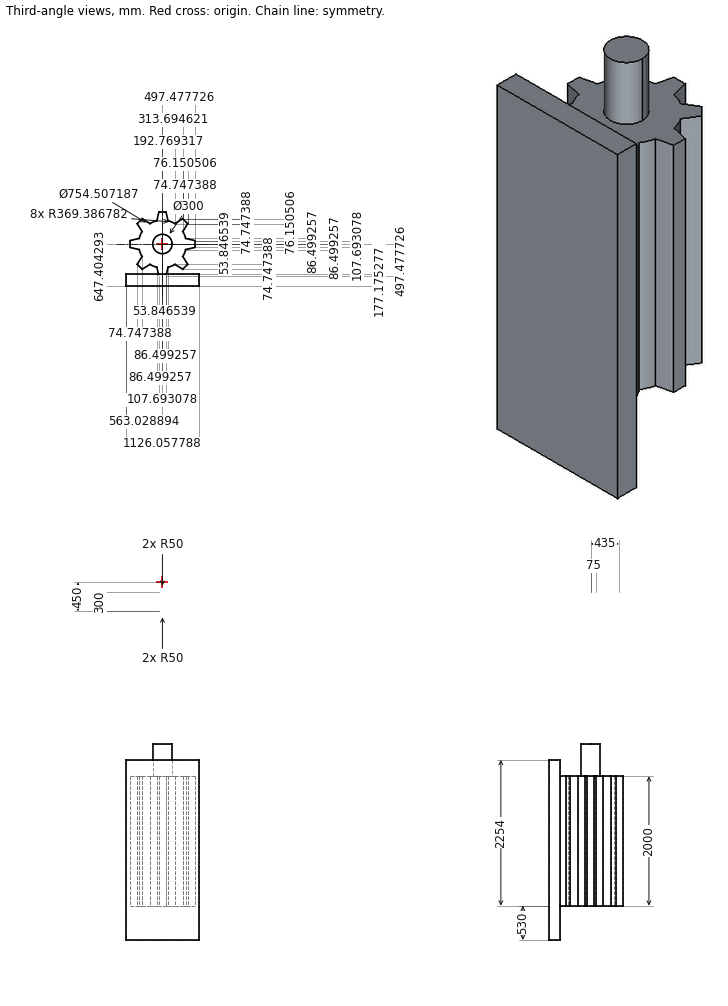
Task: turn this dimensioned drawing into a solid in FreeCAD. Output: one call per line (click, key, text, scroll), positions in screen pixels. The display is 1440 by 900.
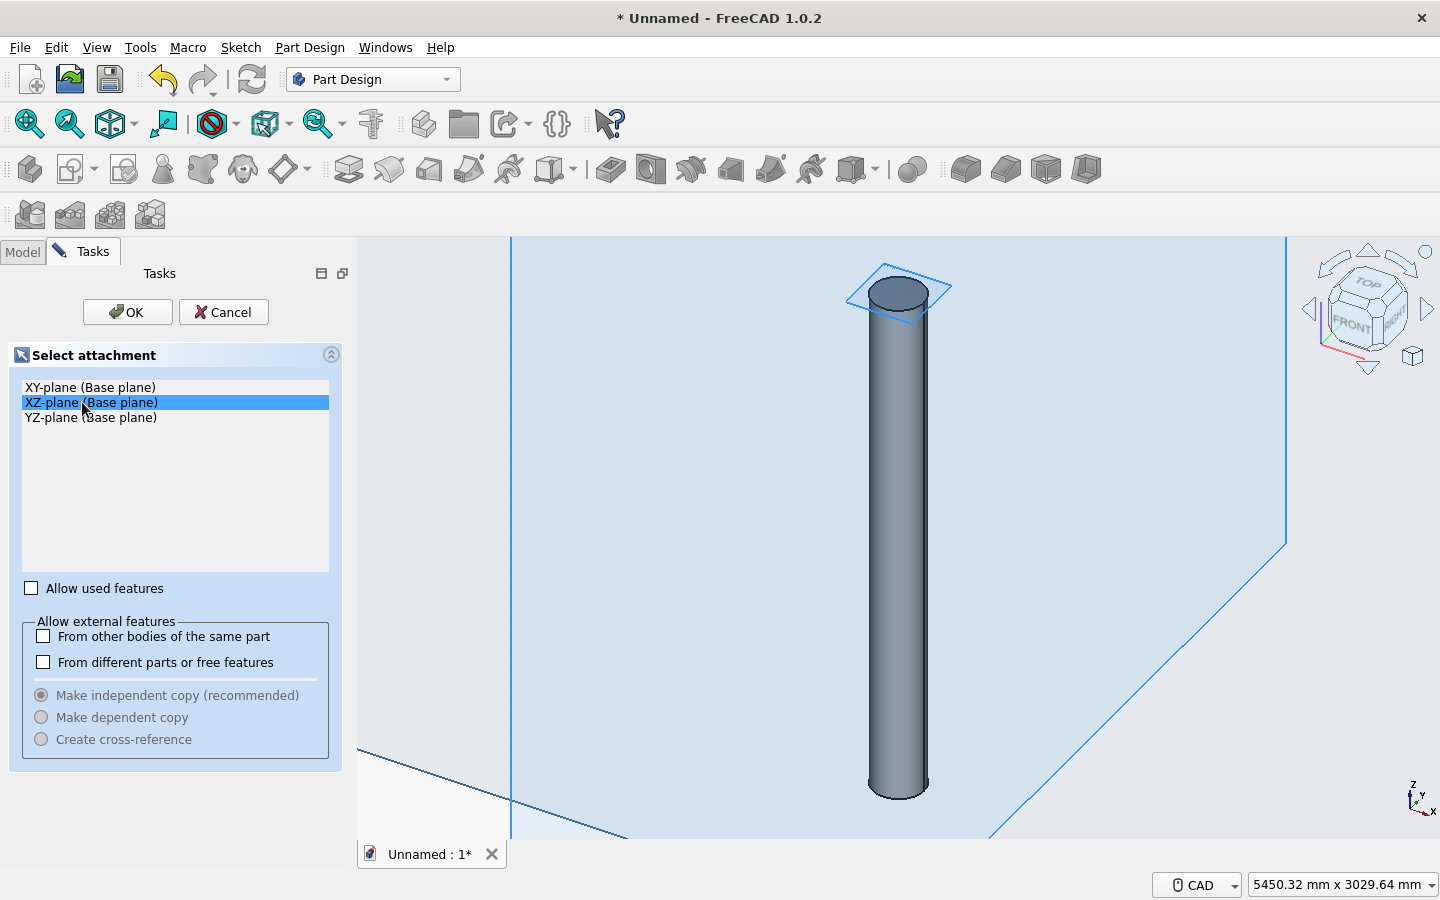
click(128, 312)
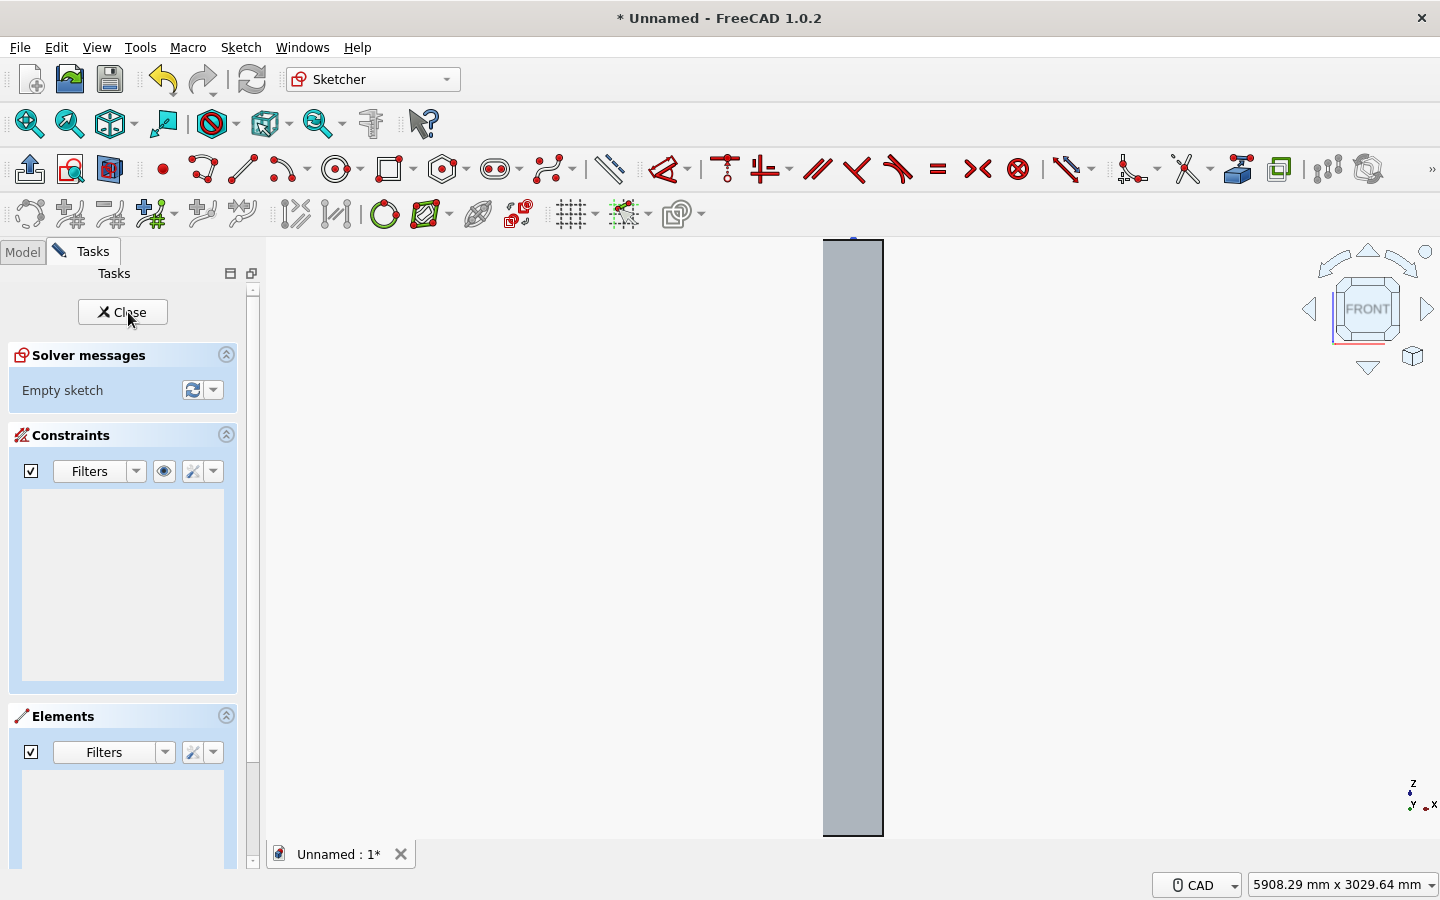
click(110, 170)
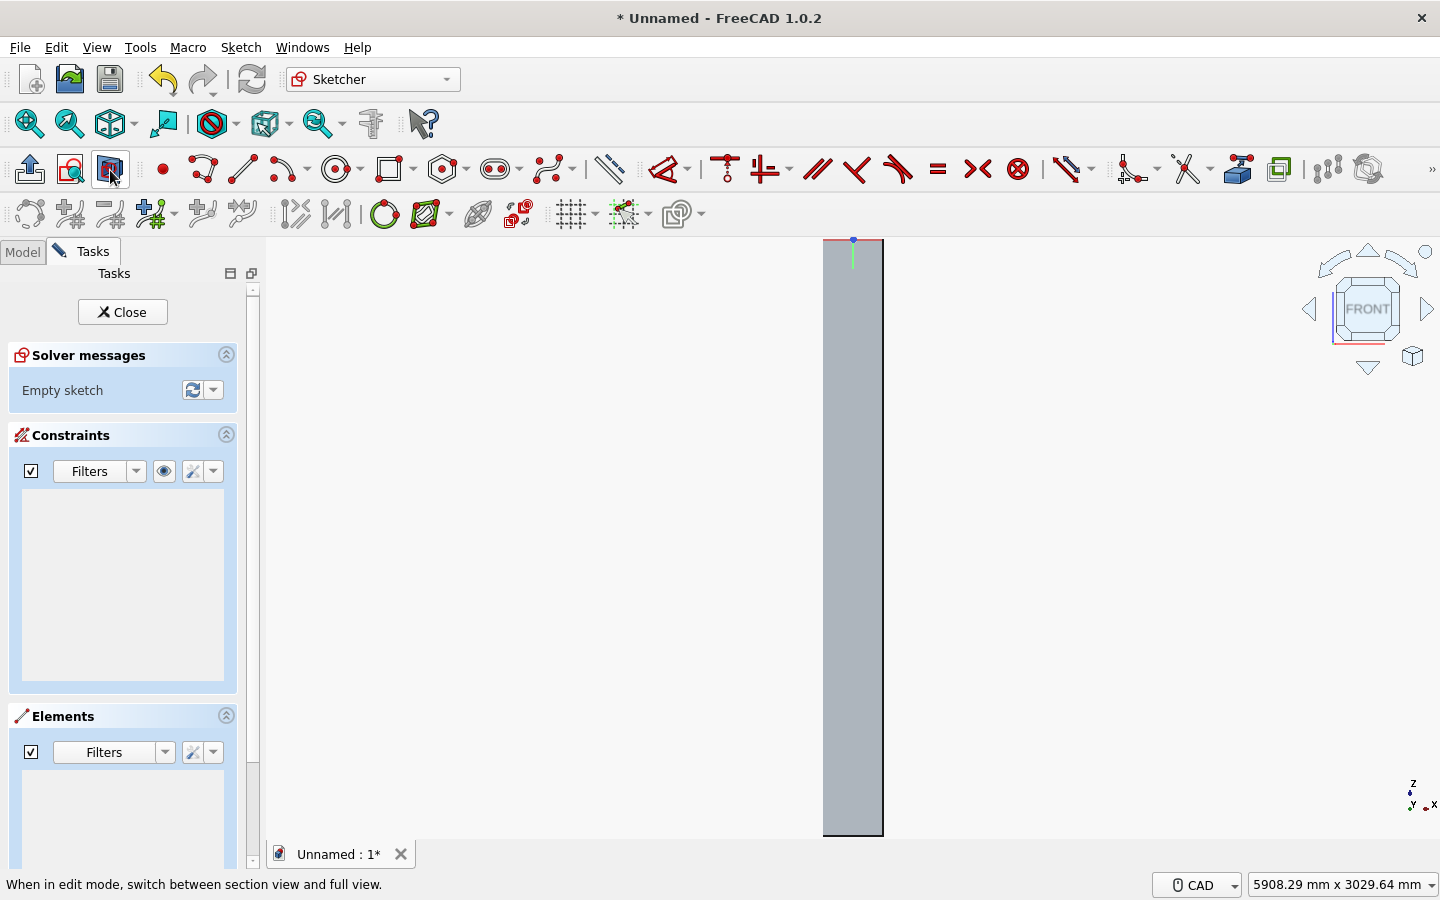
scroll(784, 538, down, 5)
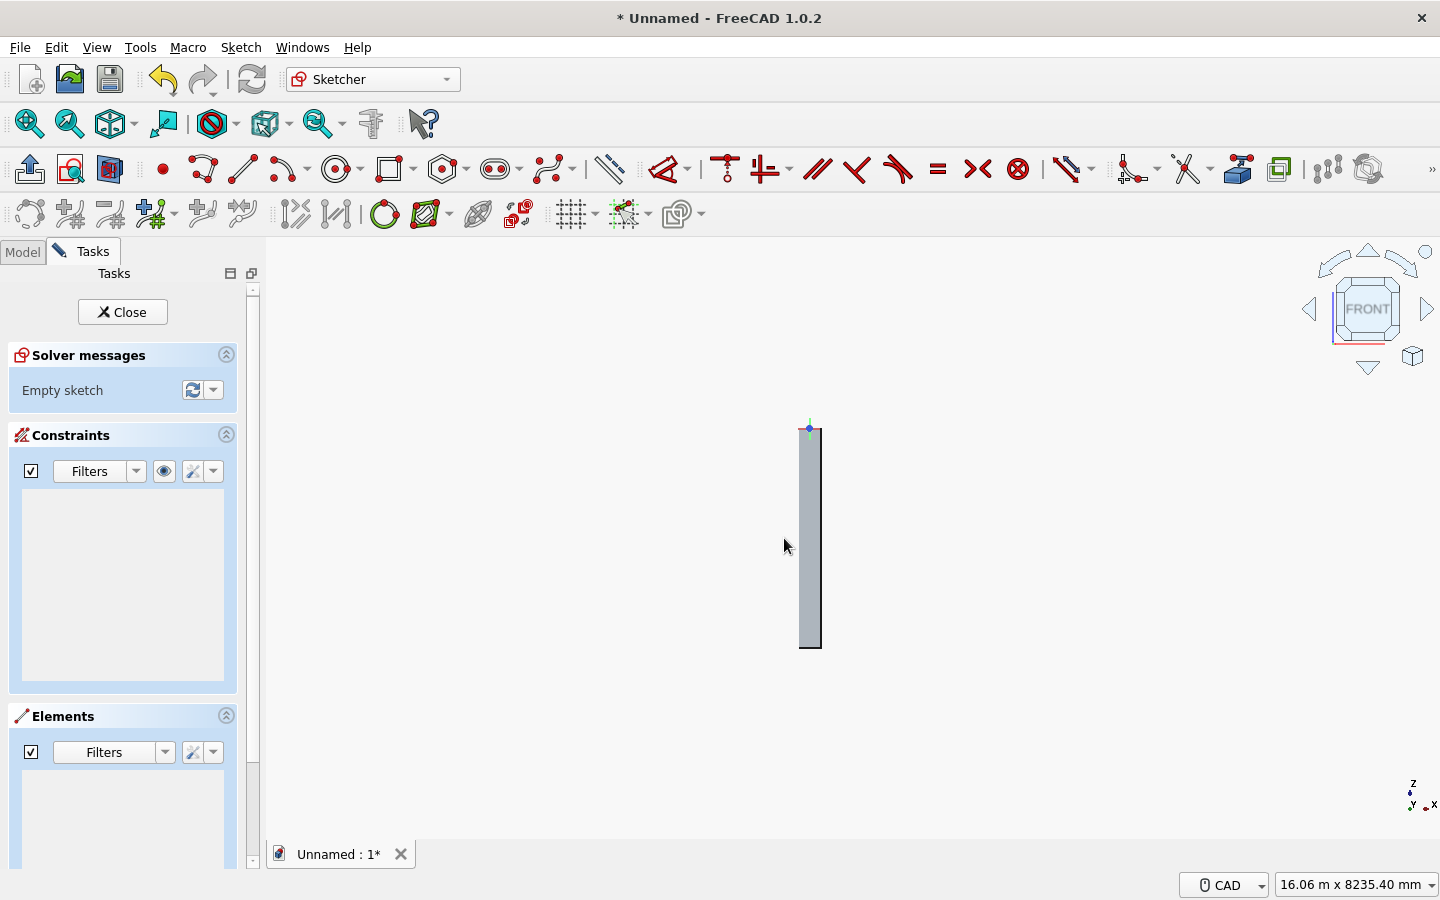
scroll(812, 438, up, 12)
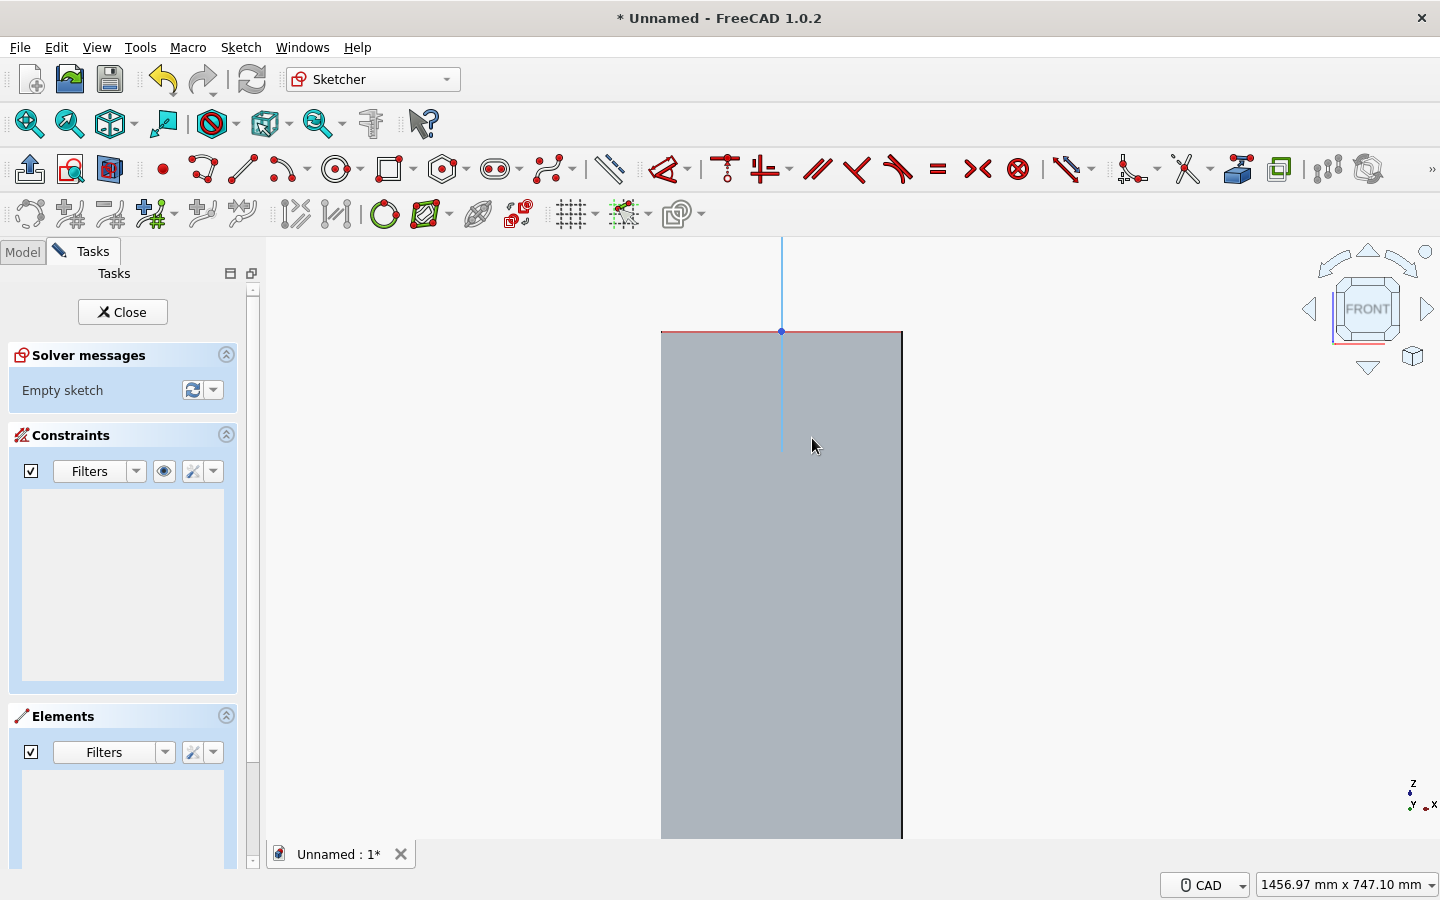
click(496, 170)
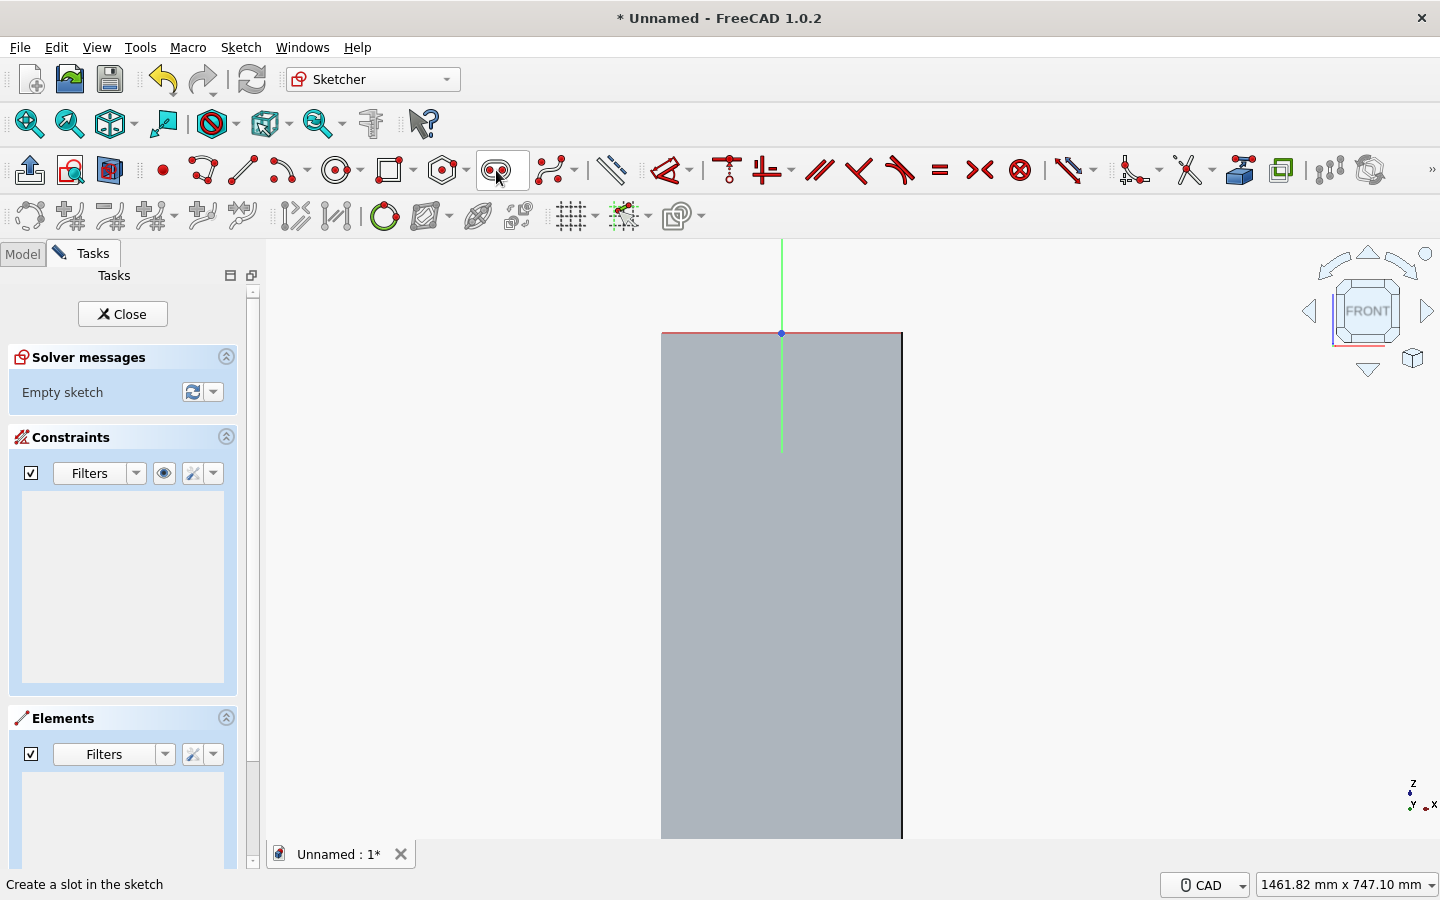
click(782, 695)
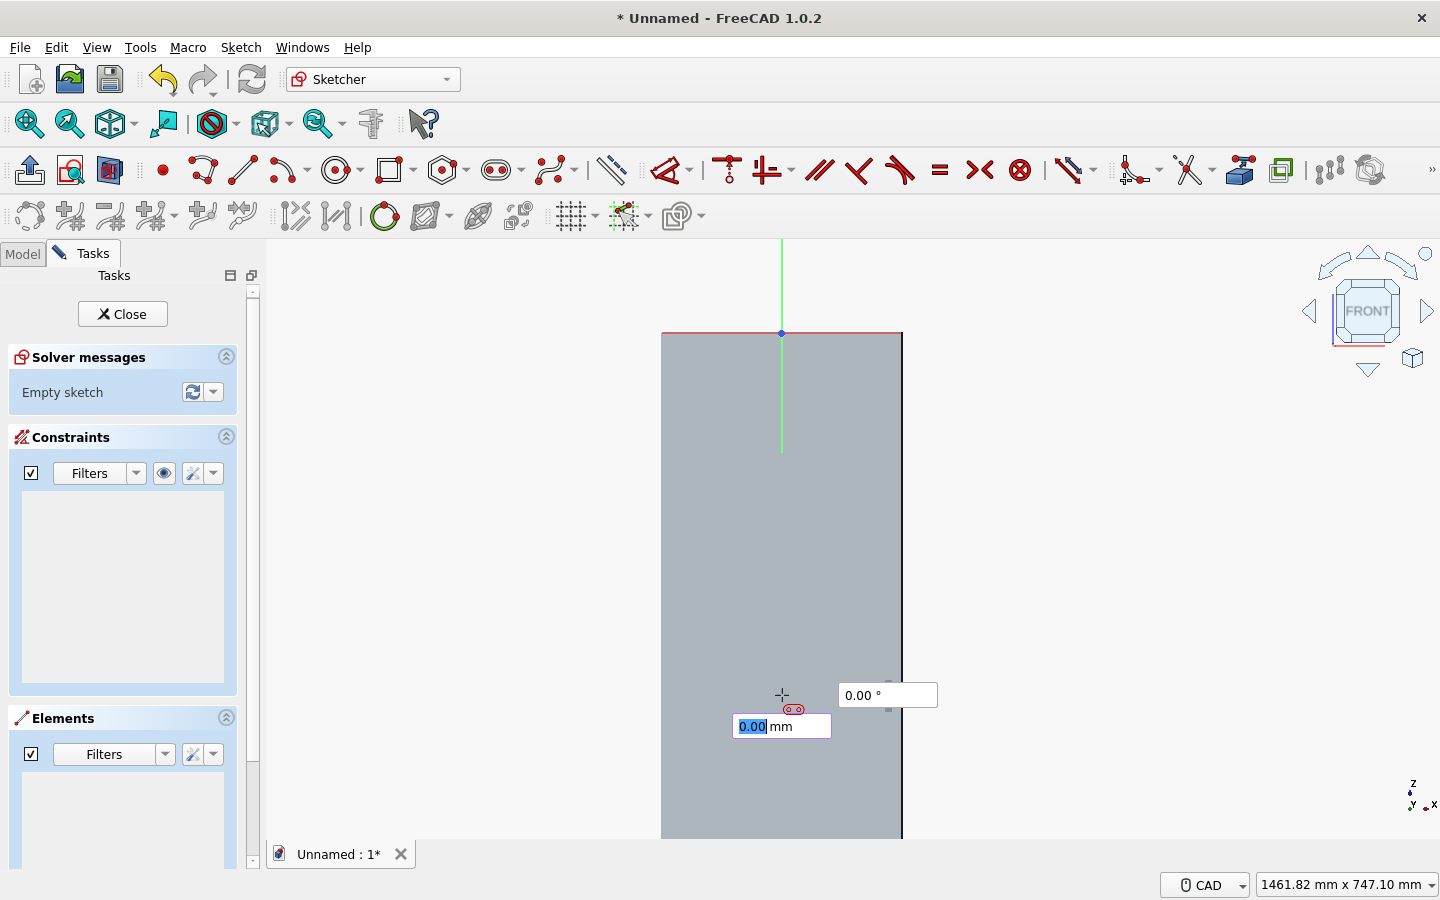
click(791, 454)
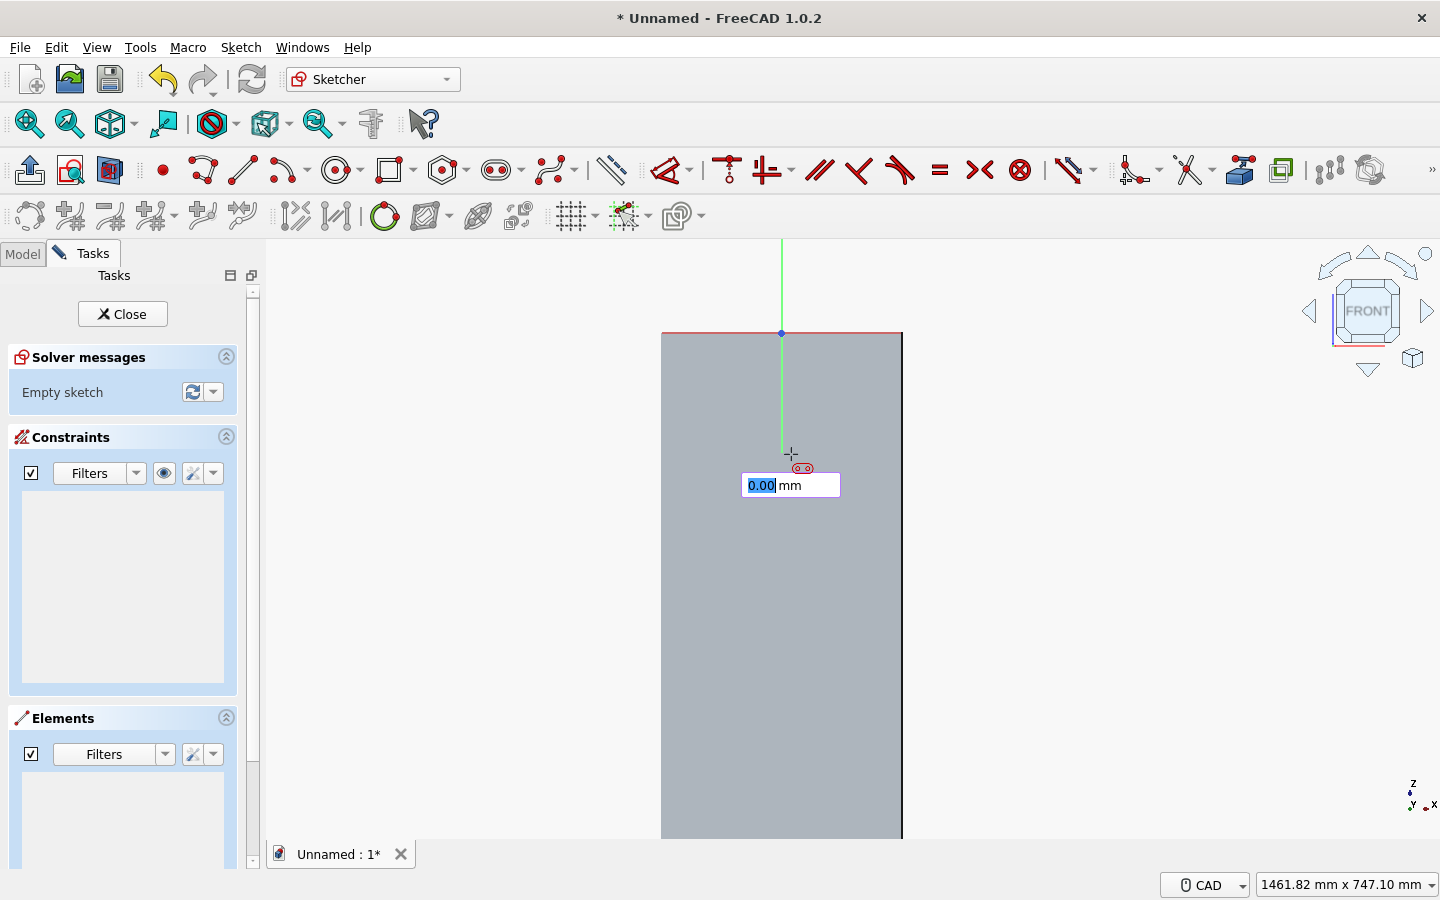
click(742, 574)
key(Escape)